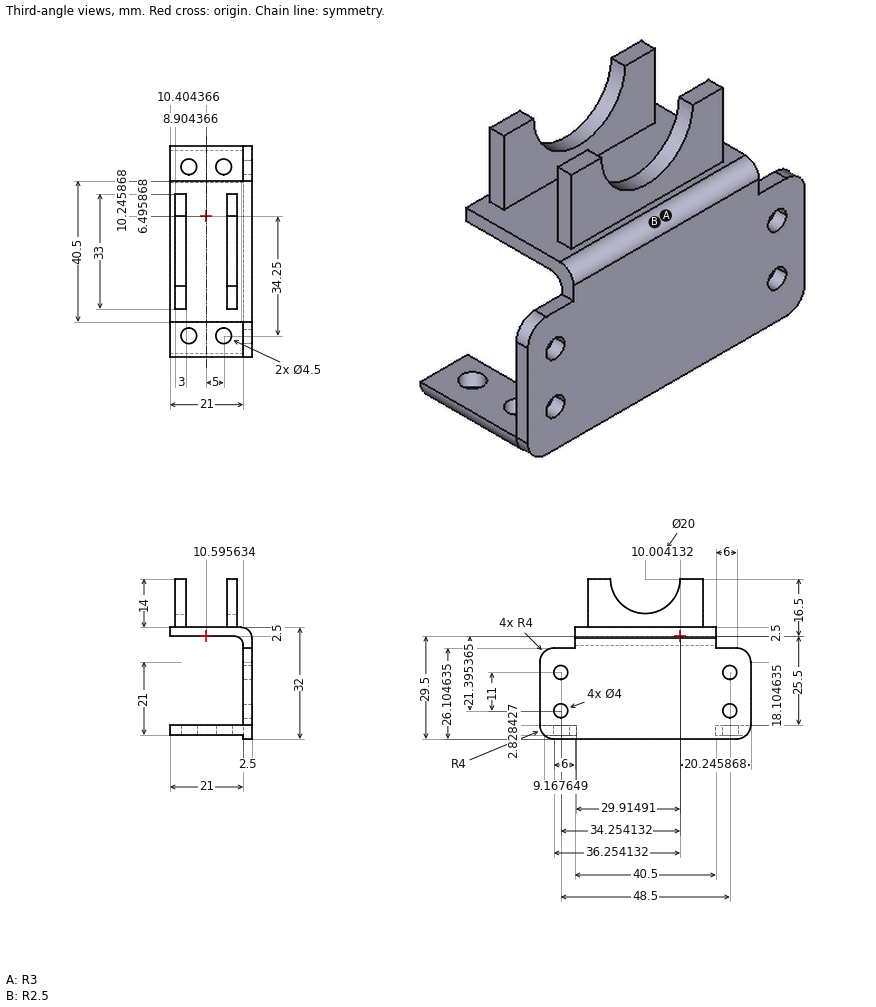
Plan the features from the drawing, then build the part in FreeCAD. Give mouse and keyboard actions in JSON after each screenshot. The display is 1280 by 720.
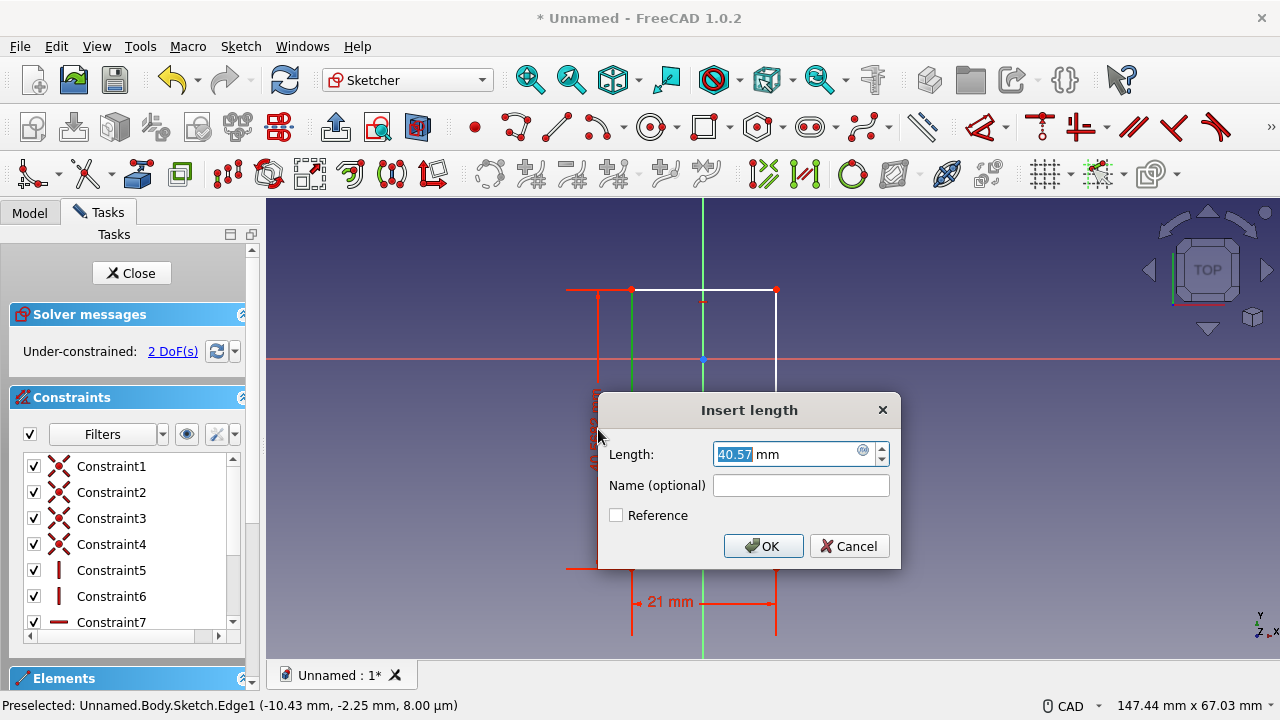
{"action": "type", "text": "40.5"}
{"action": "key", "text": "Return"}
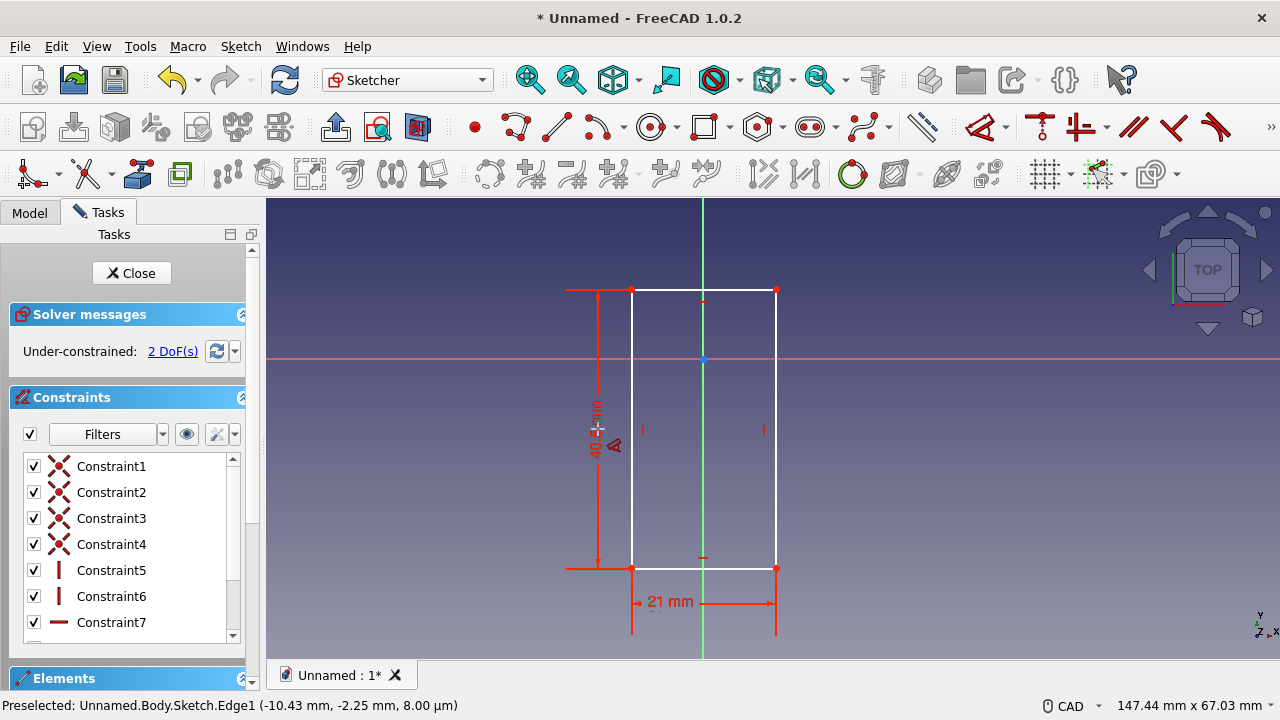
{"action": "left_click", "coordinate": [632, 290]}
{"action": "left_click", "coordinate": [667, 256]}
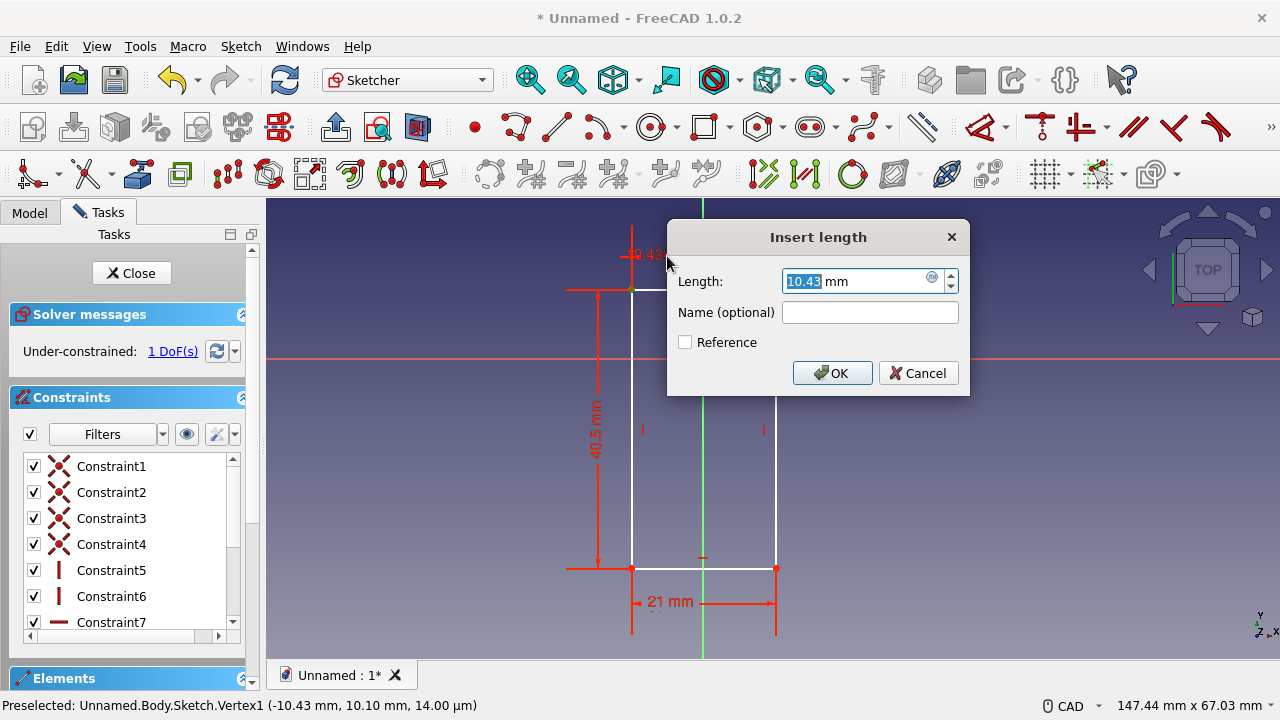
{"action": "type", "text": "10.404366"}
{"action": "key", "text": "Return"}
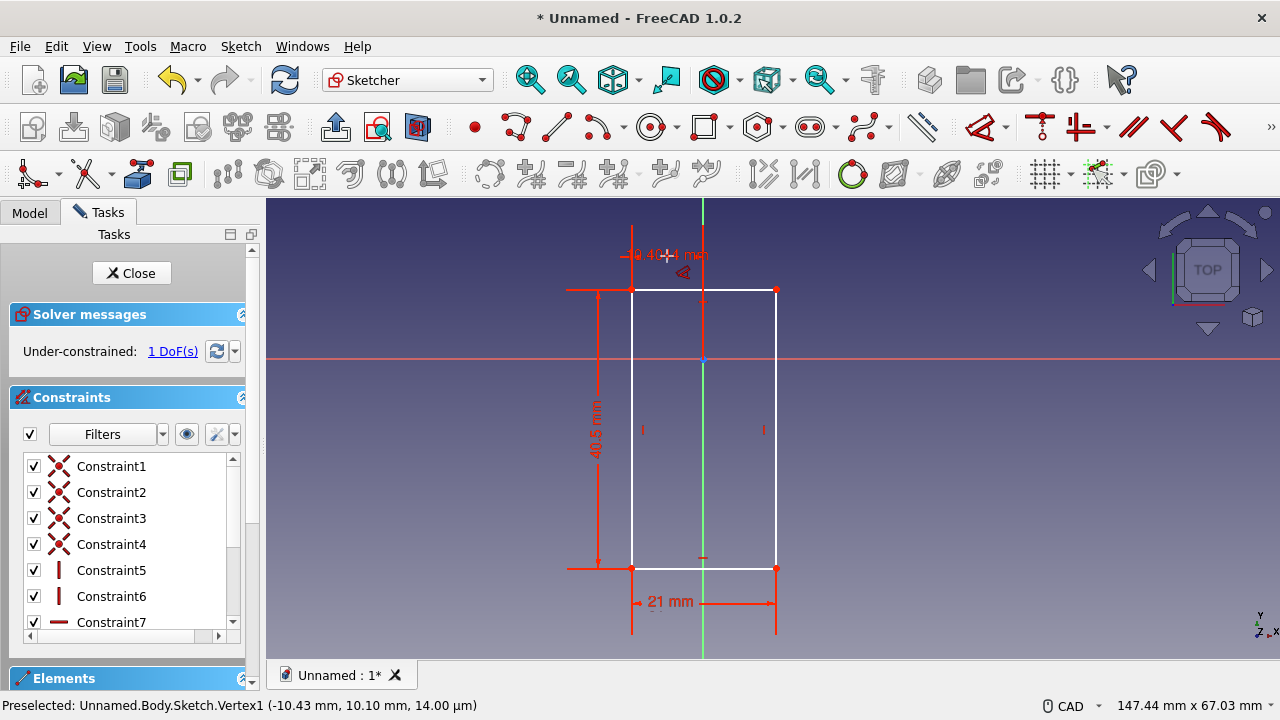
{"action": "left_click", "coordinate": [632, 290]}
{"action": "left_click", "coordinate": [598, 325]}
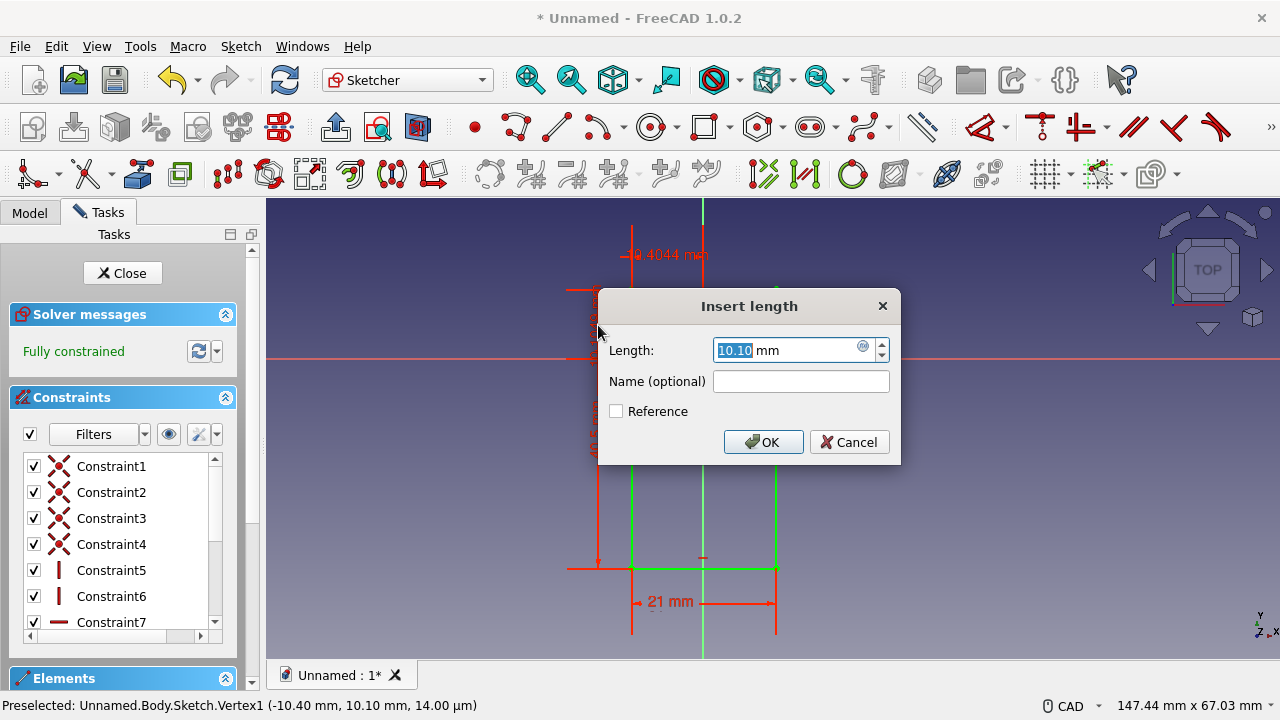
{"action": "type", "text": "10.245868"}
{"action": "key", "text": "Return"}
{"action": "key", "text": "Escape"}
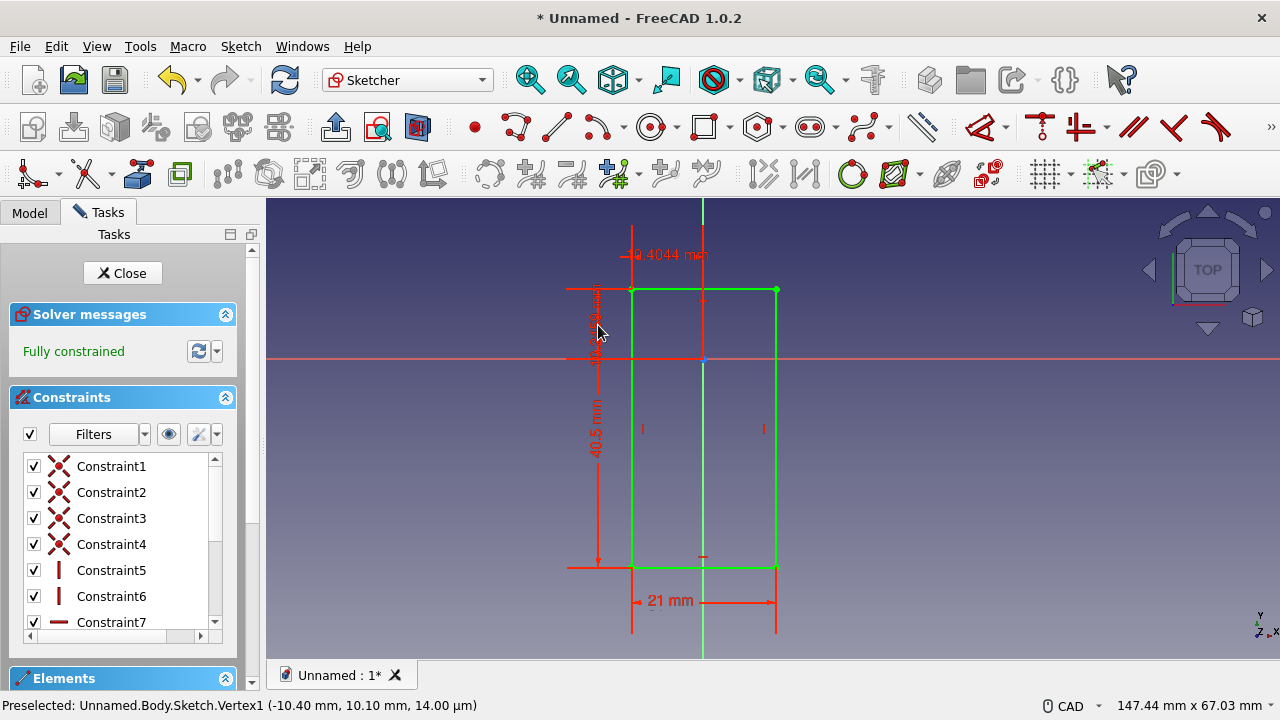
{"action": "left_click", "coordinate": [123, 273]}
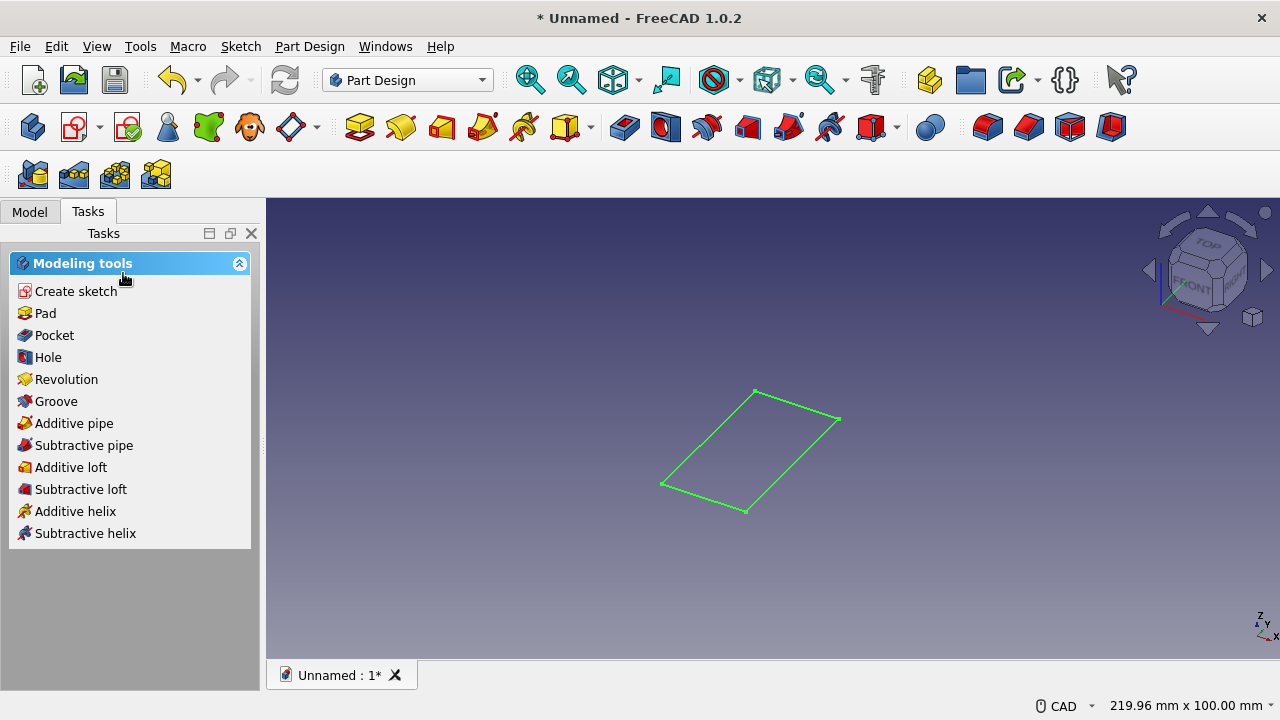
{"action": "left_click", "coordinate": [360, 128]}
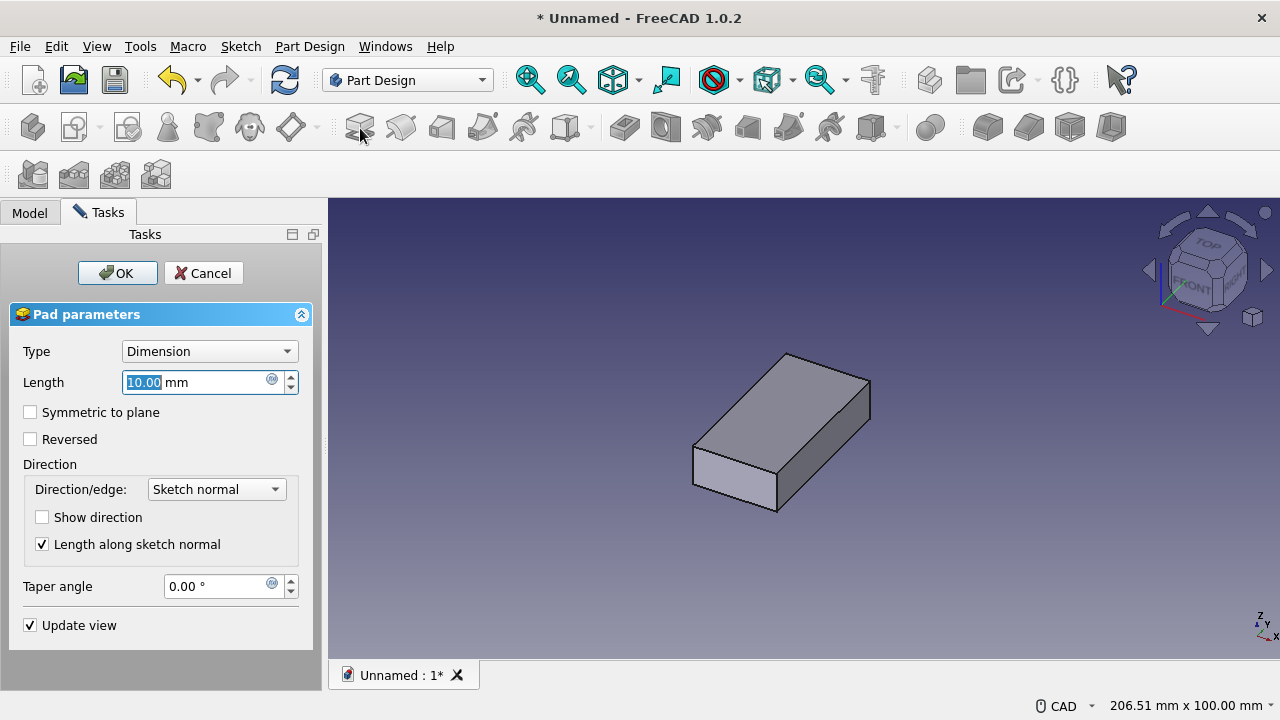
{"action": "type", "text": "2.5"}
{"action": "key", "text": "Tab"}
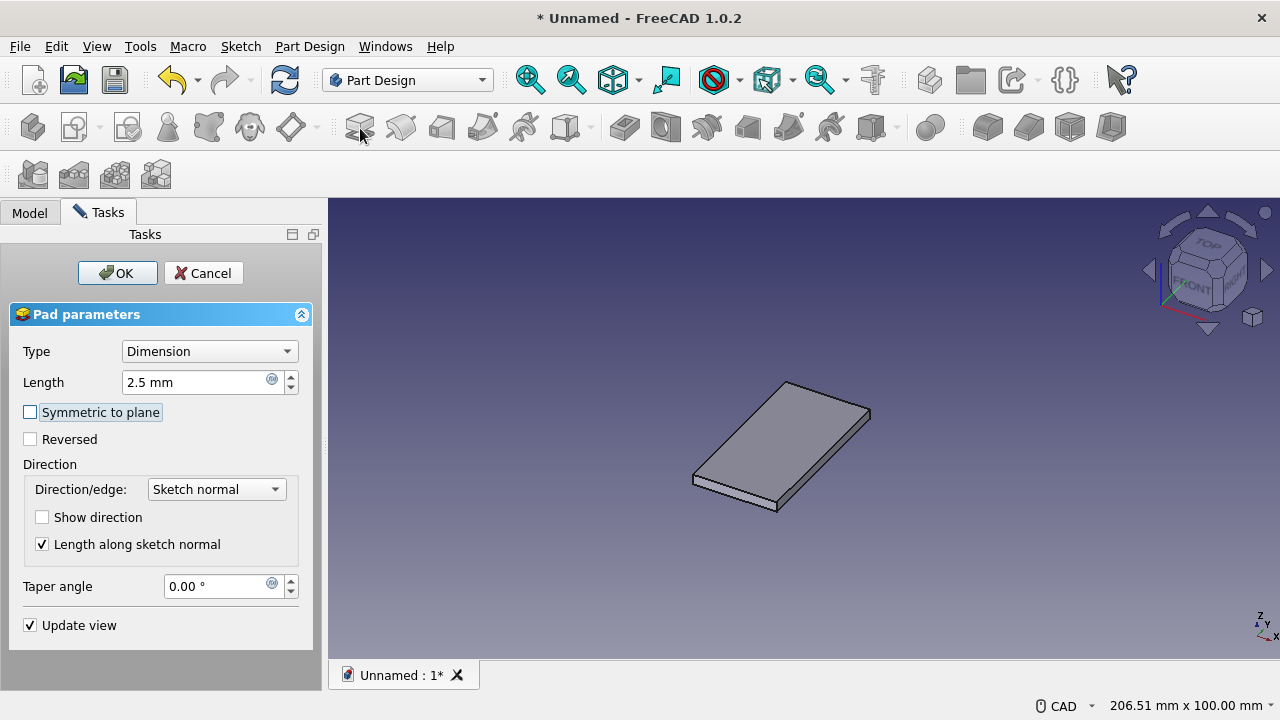
{"action": "left_click", "coordinate": [118, 273]}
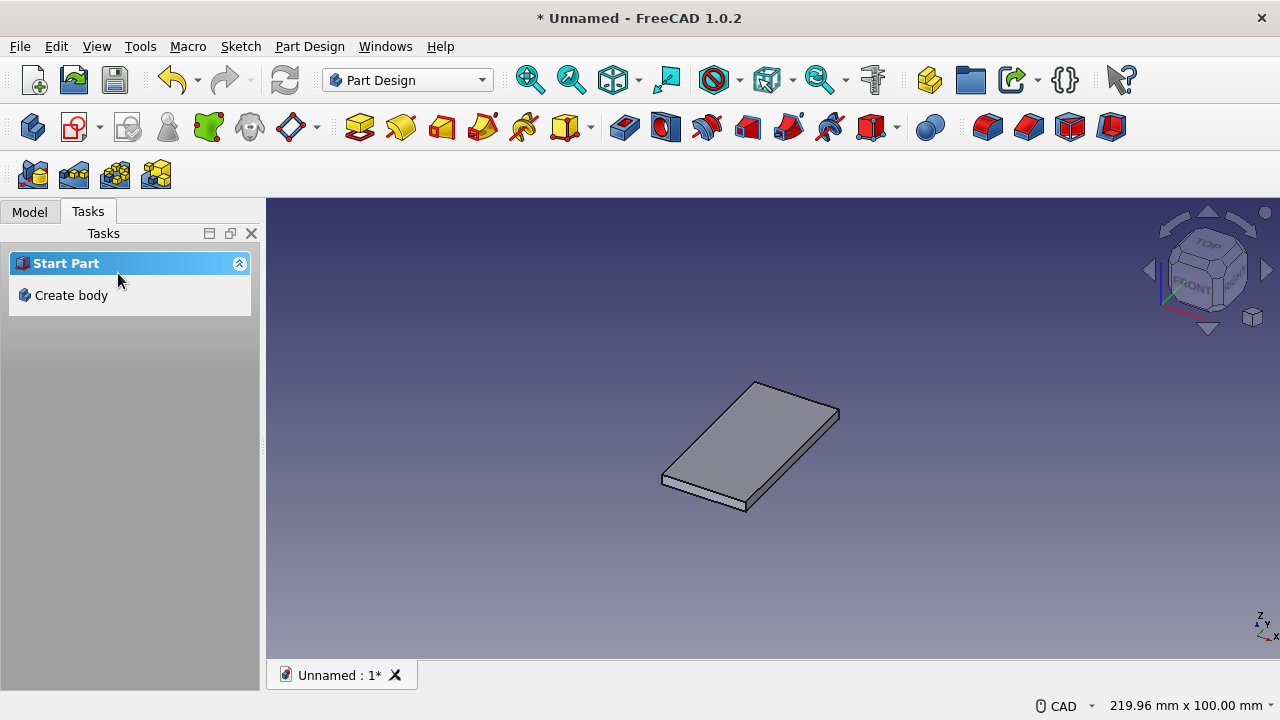
{"action": "left_click", "coordinate": [531, 80]}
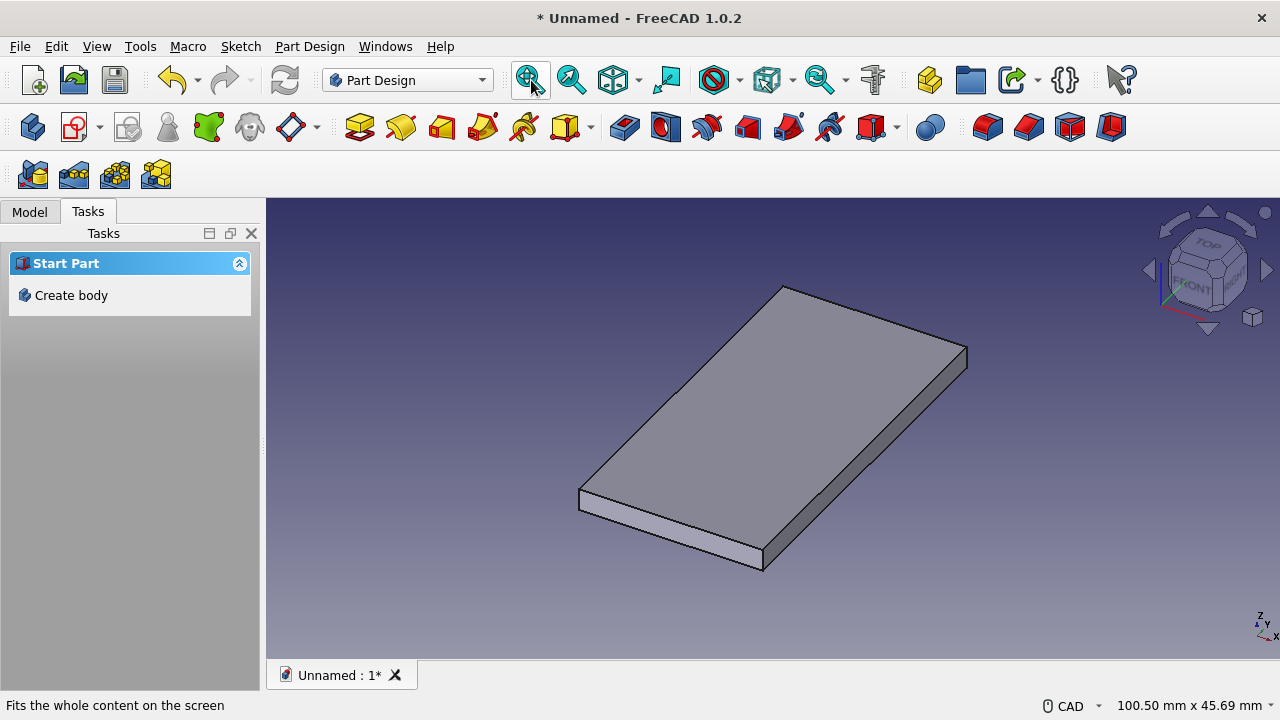
{"action": "left_click", "coordinate": [802, 388]}